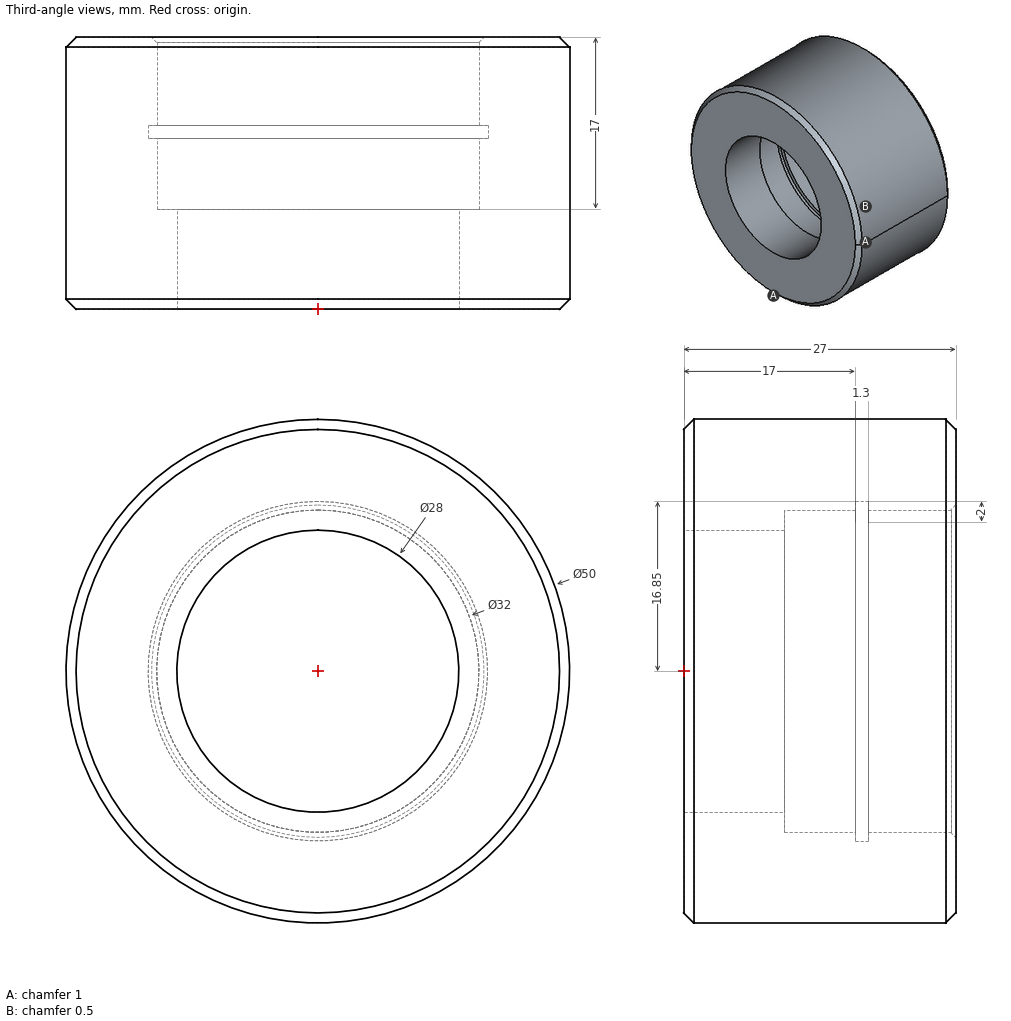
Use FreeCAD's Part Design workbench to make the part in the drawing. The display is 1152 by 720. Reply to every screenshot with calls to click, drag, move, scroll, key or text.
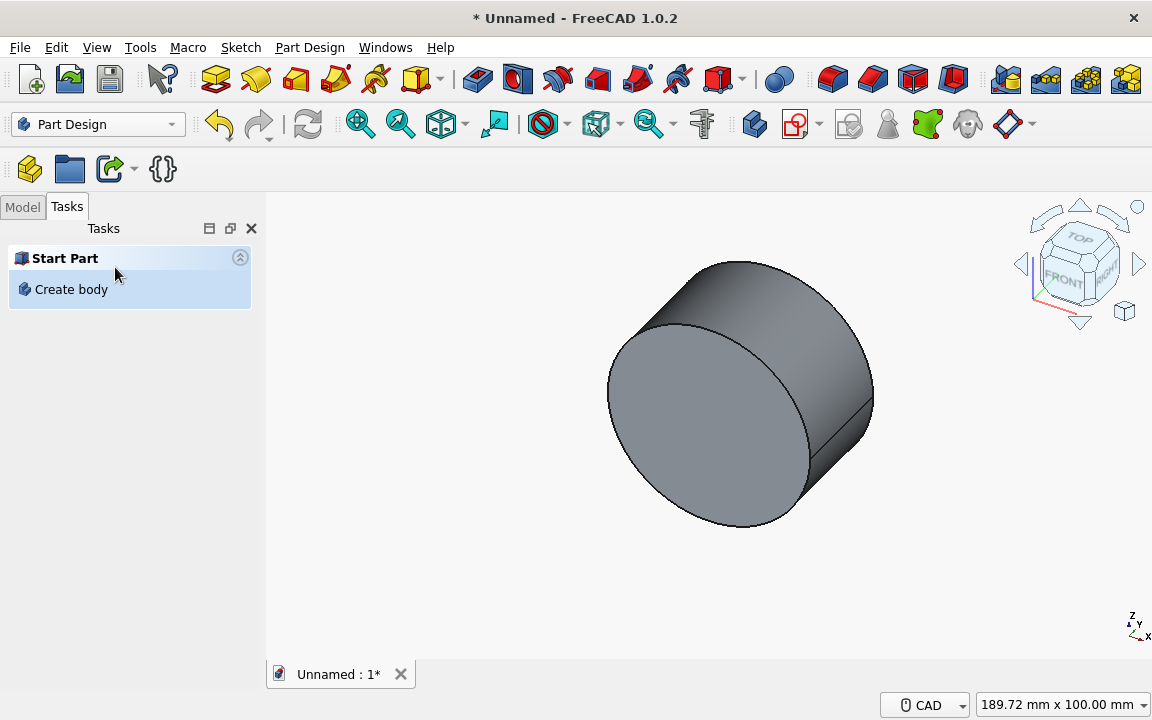
key(4)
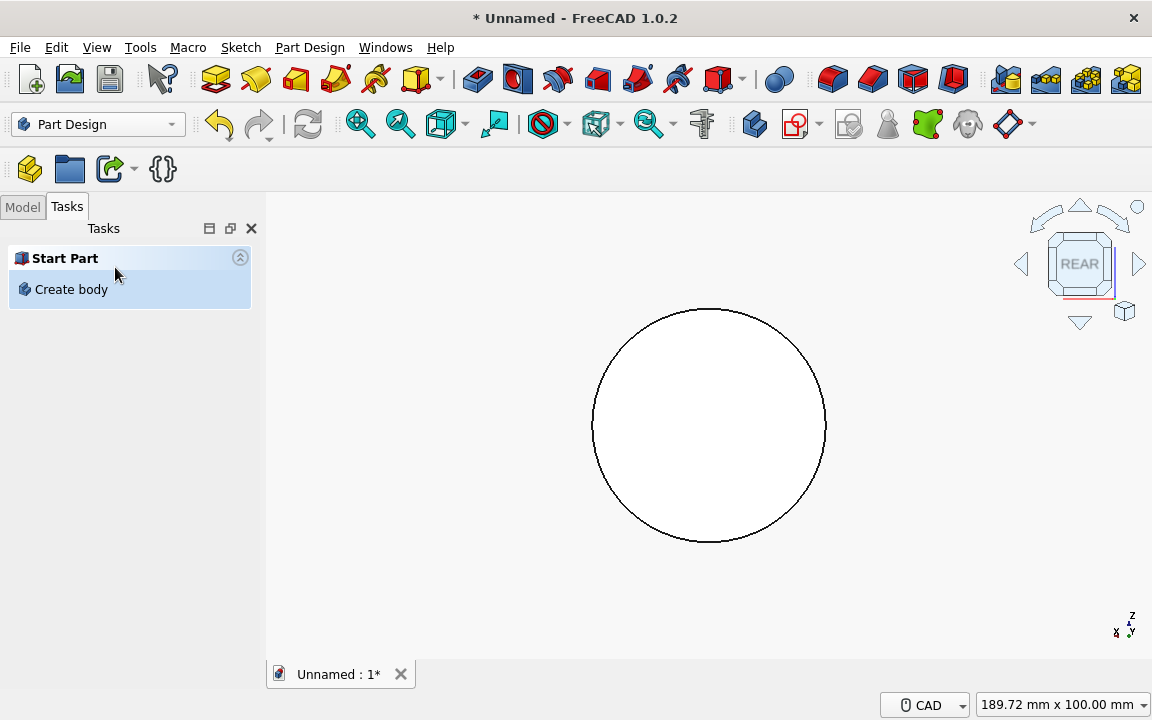
click(709, 424)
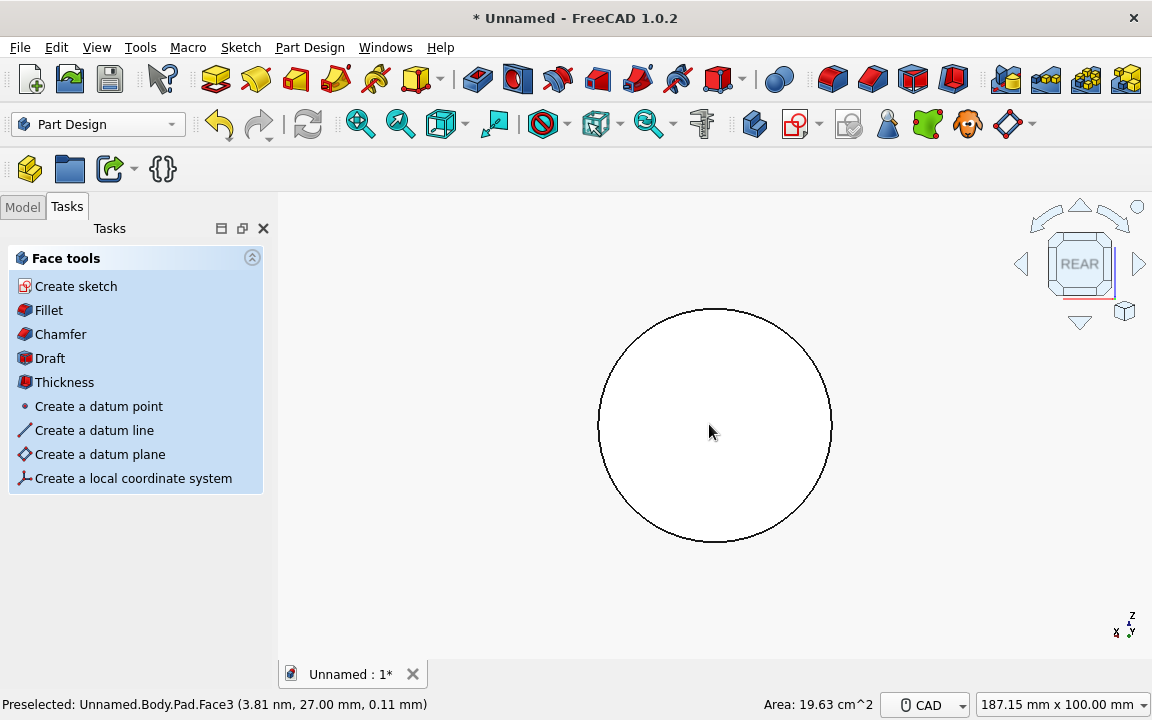
click(796, 124)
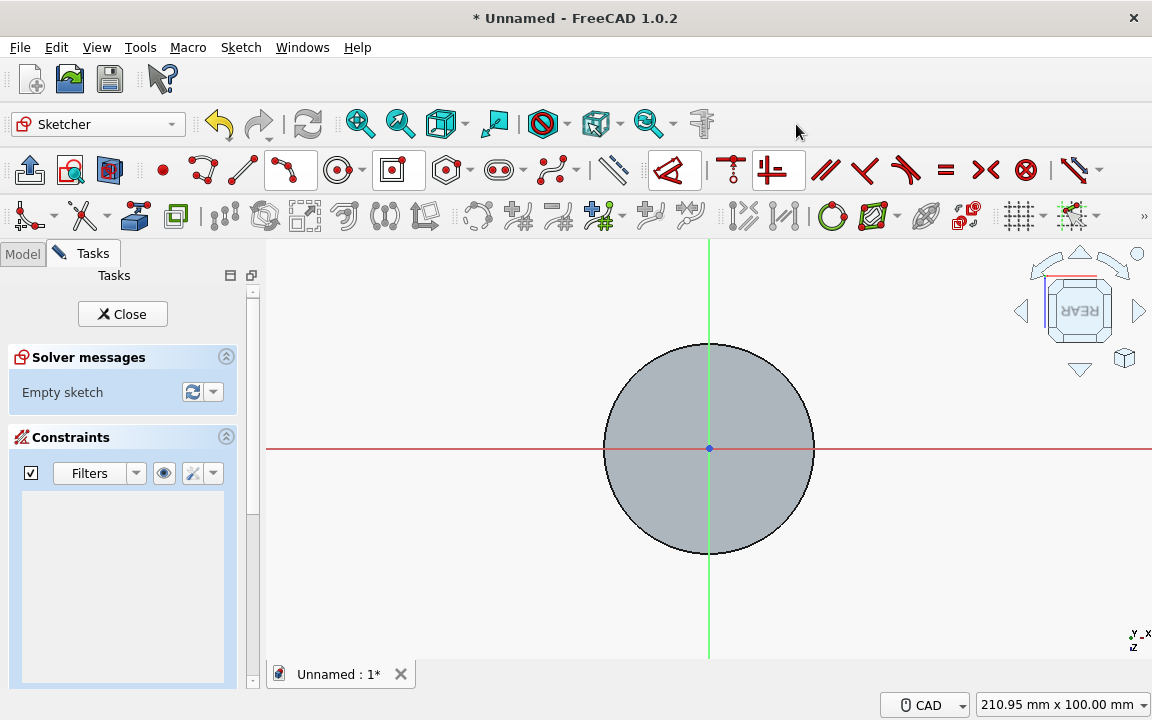
scroll(792, 449, up, 3)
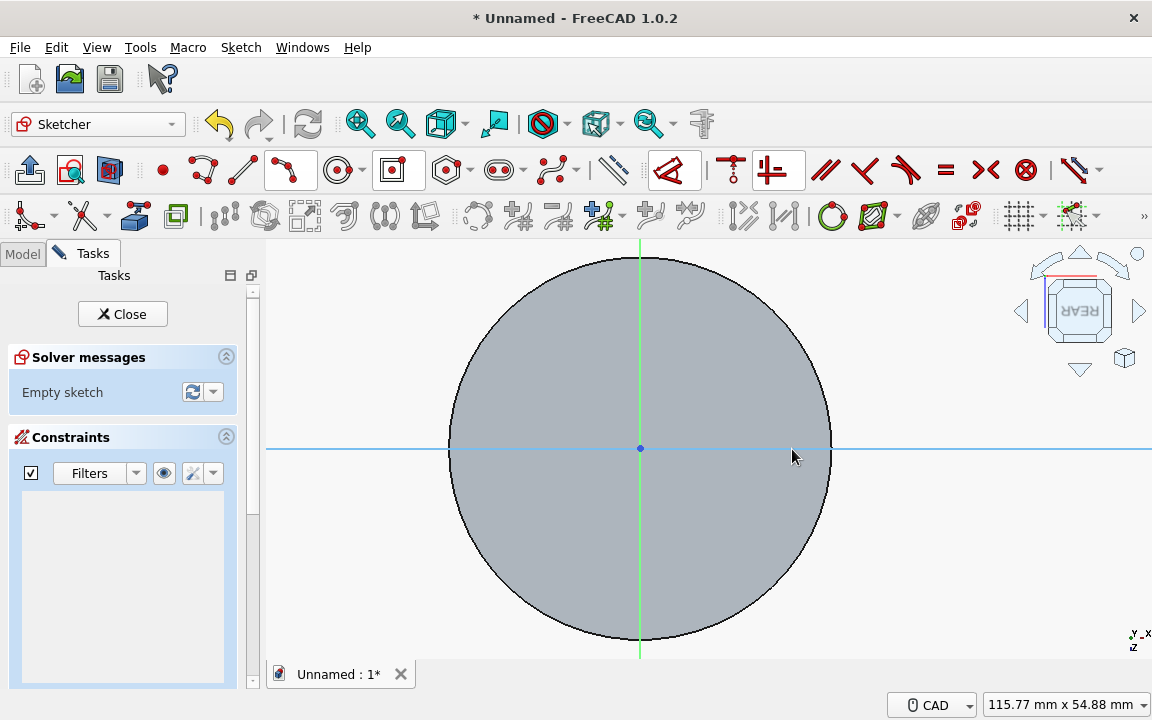
click(338, 170)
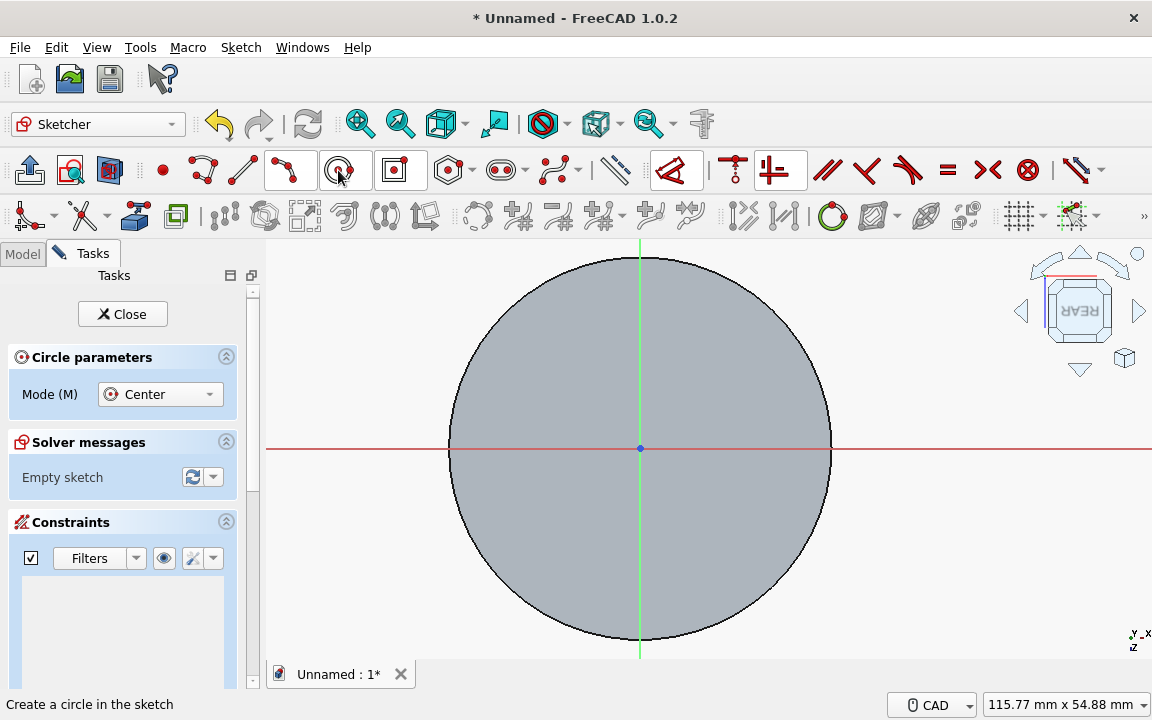
click(640, 449)
move(727, 362)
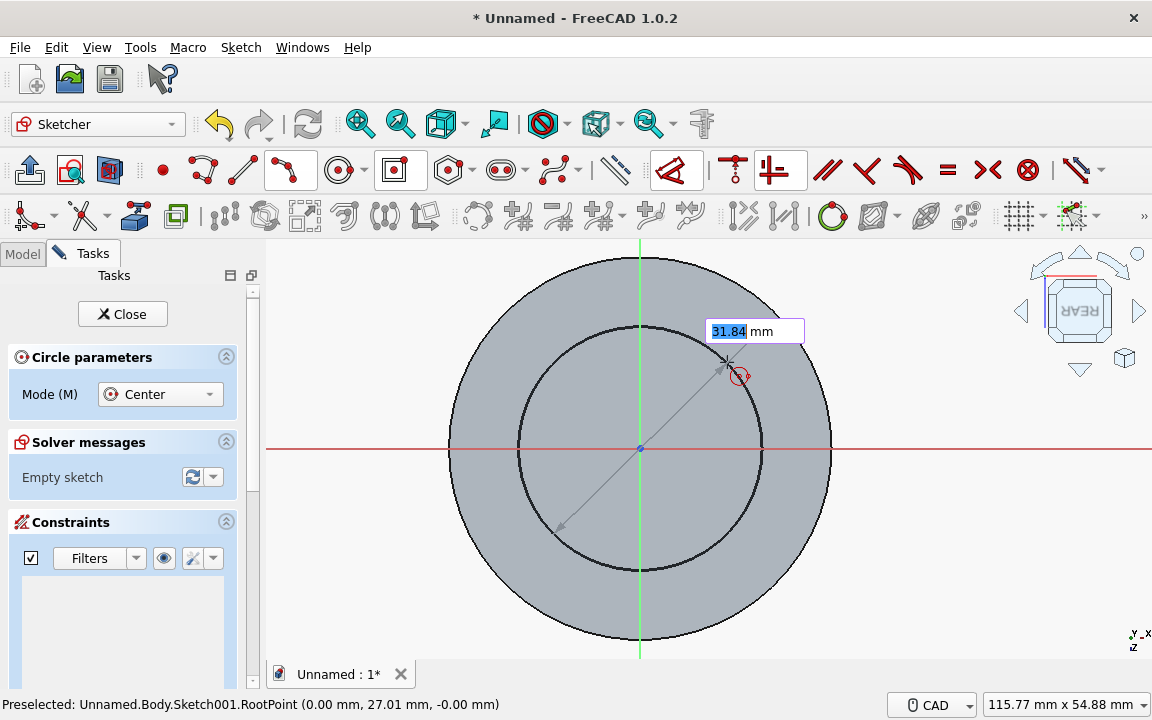
text(32)
key(Return)
key(Escape)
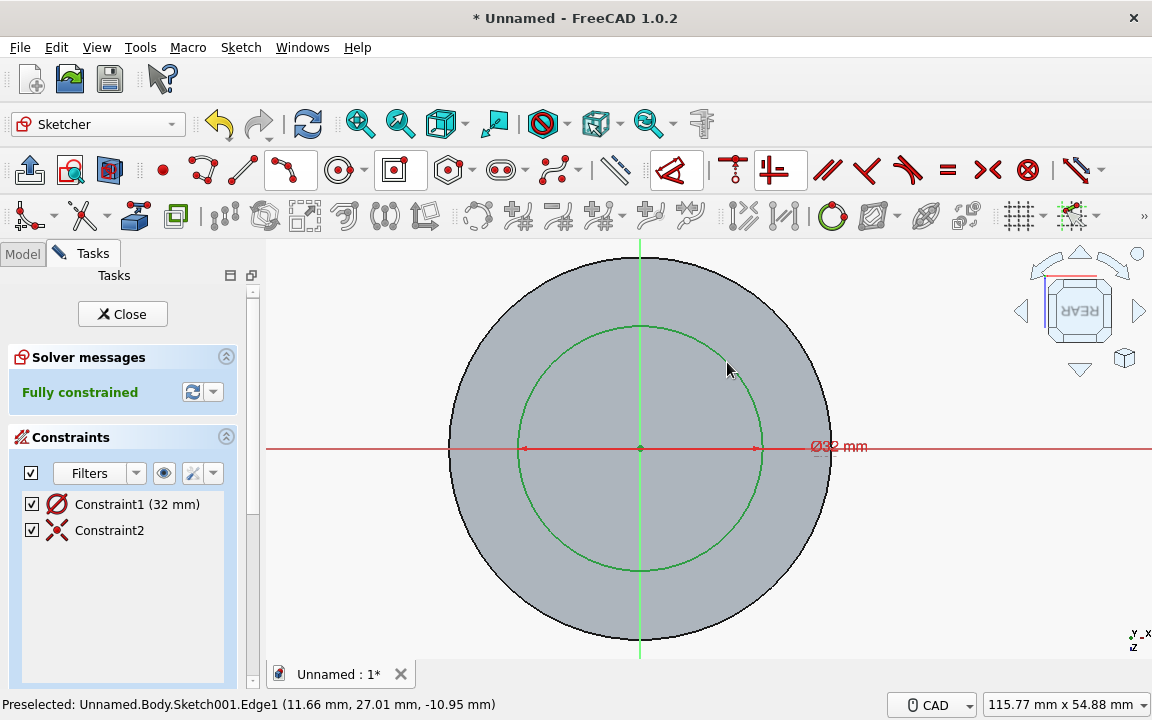
click(123, 314)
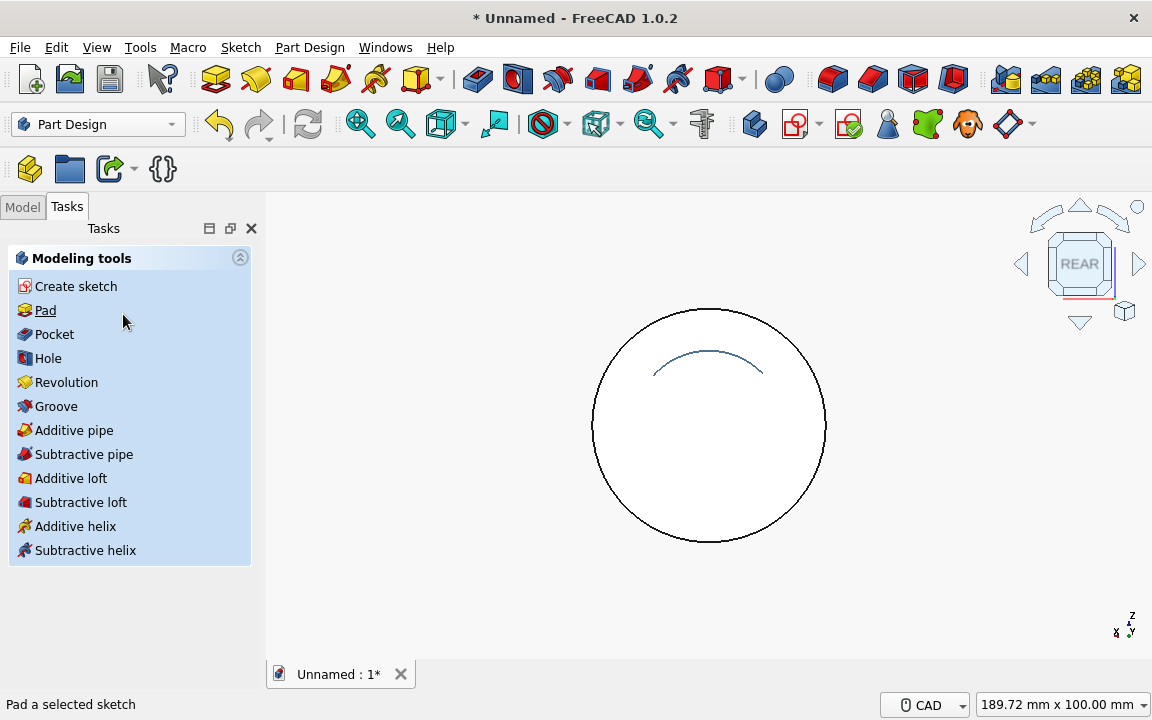
click(478, 80)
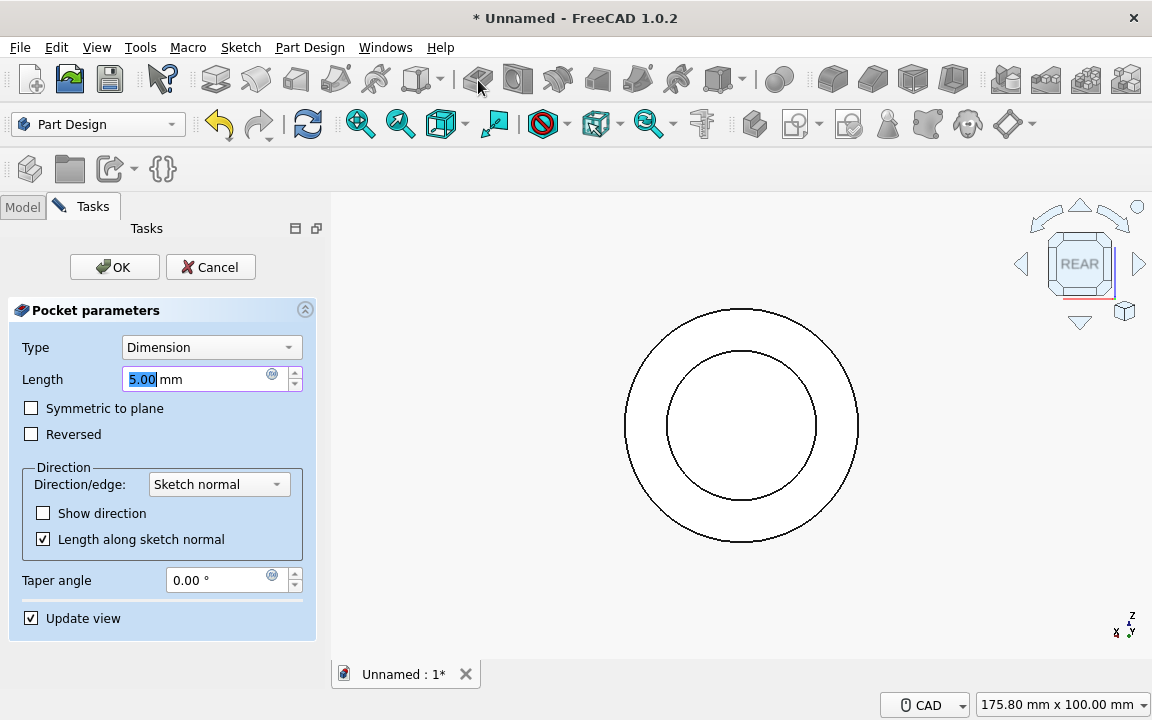
text(17)
key(Tab)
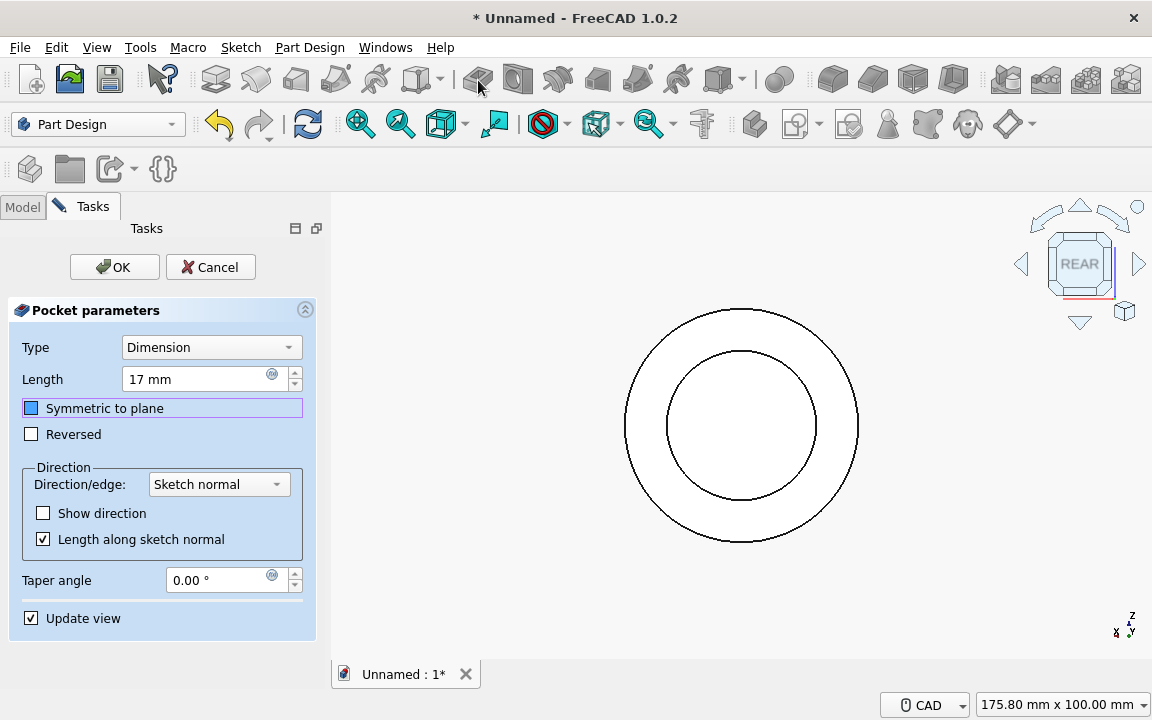
click(115, 267)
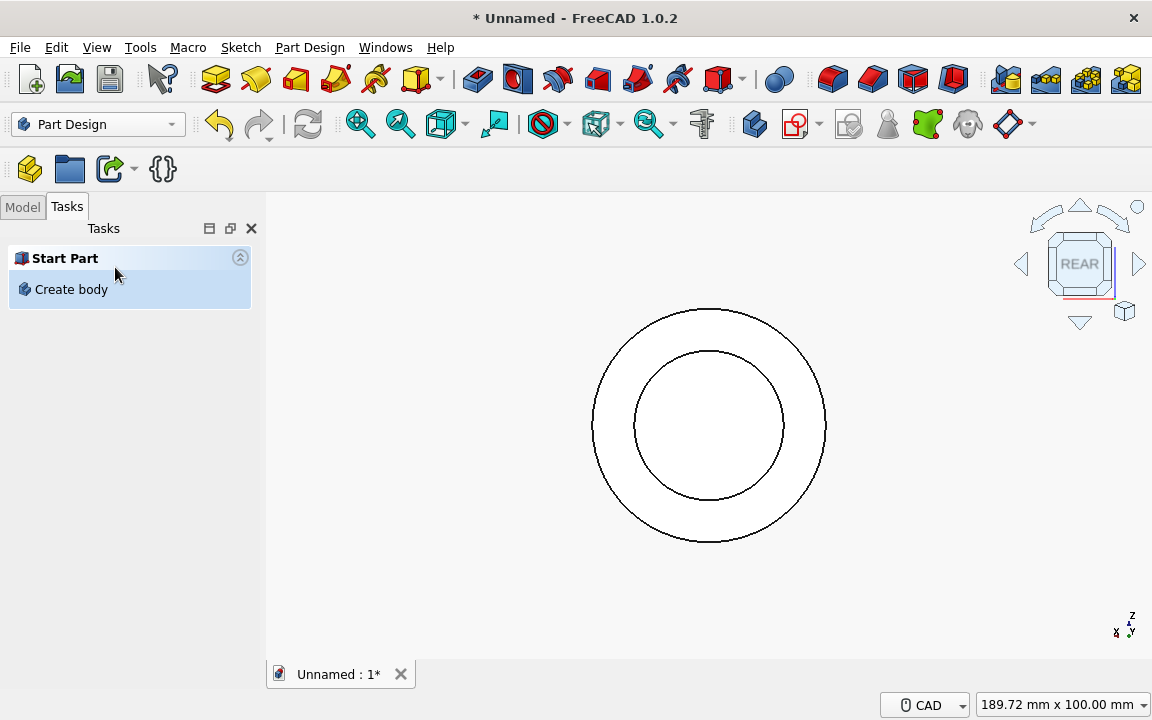
click(709, 424)